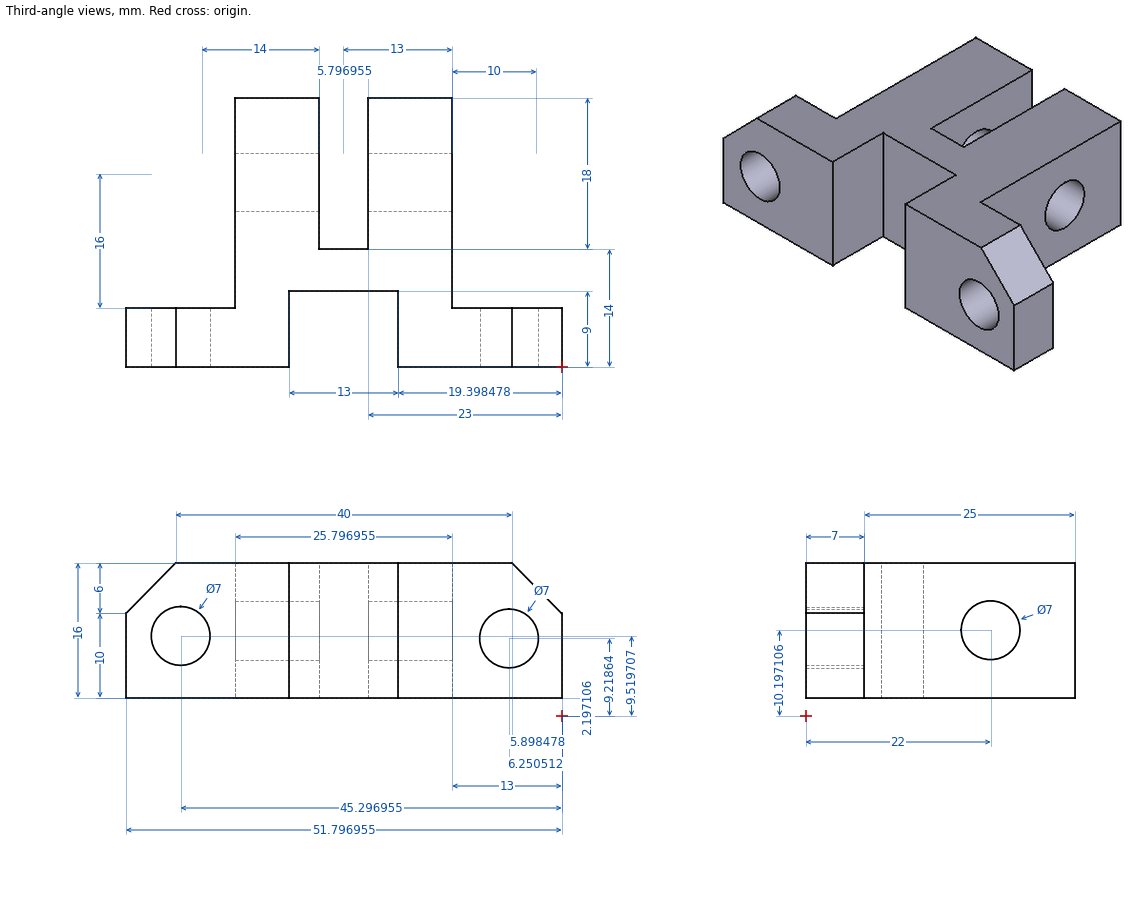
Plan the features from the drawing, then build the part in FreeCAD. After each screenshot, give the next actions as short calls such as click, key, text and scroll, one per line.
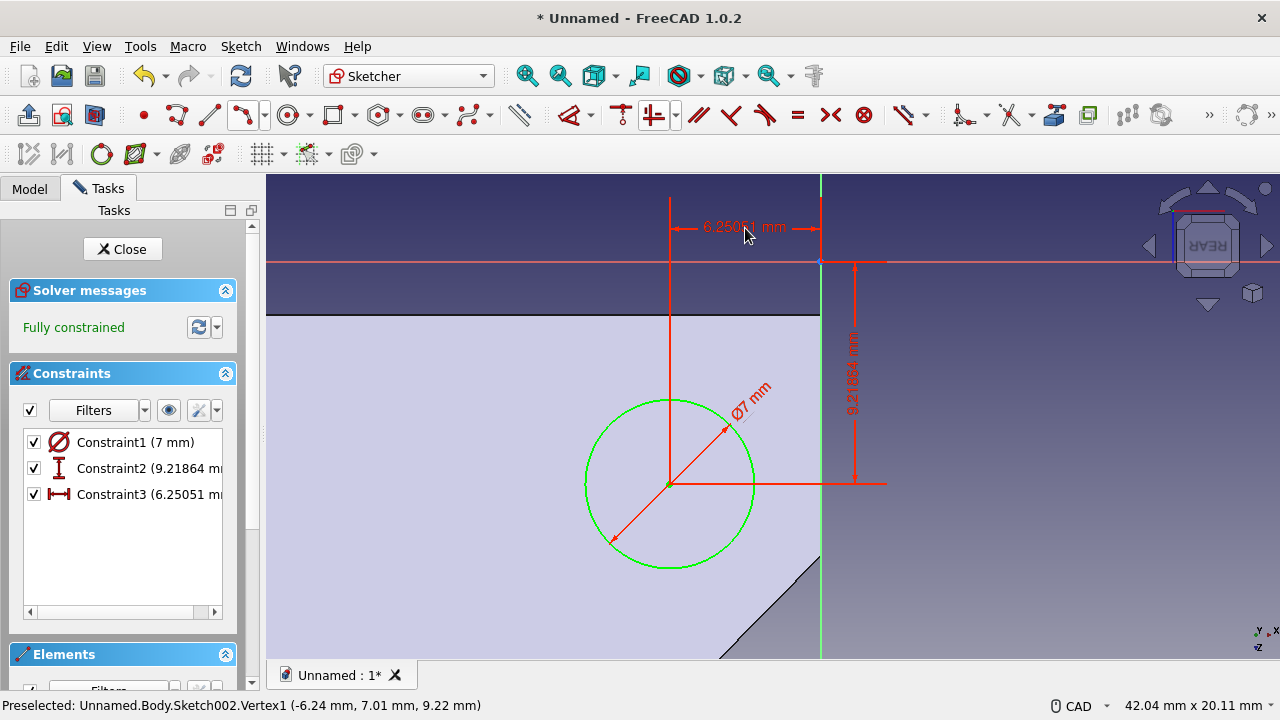
click(123, 249)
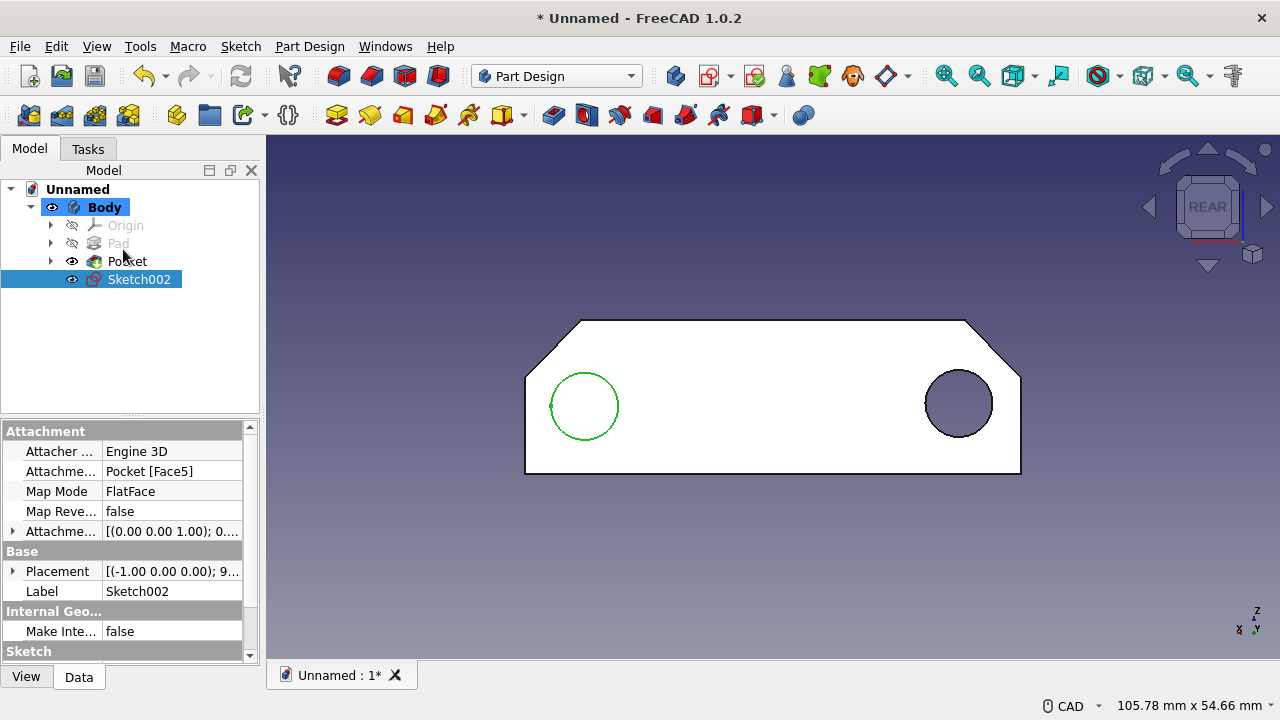
click(554, 116)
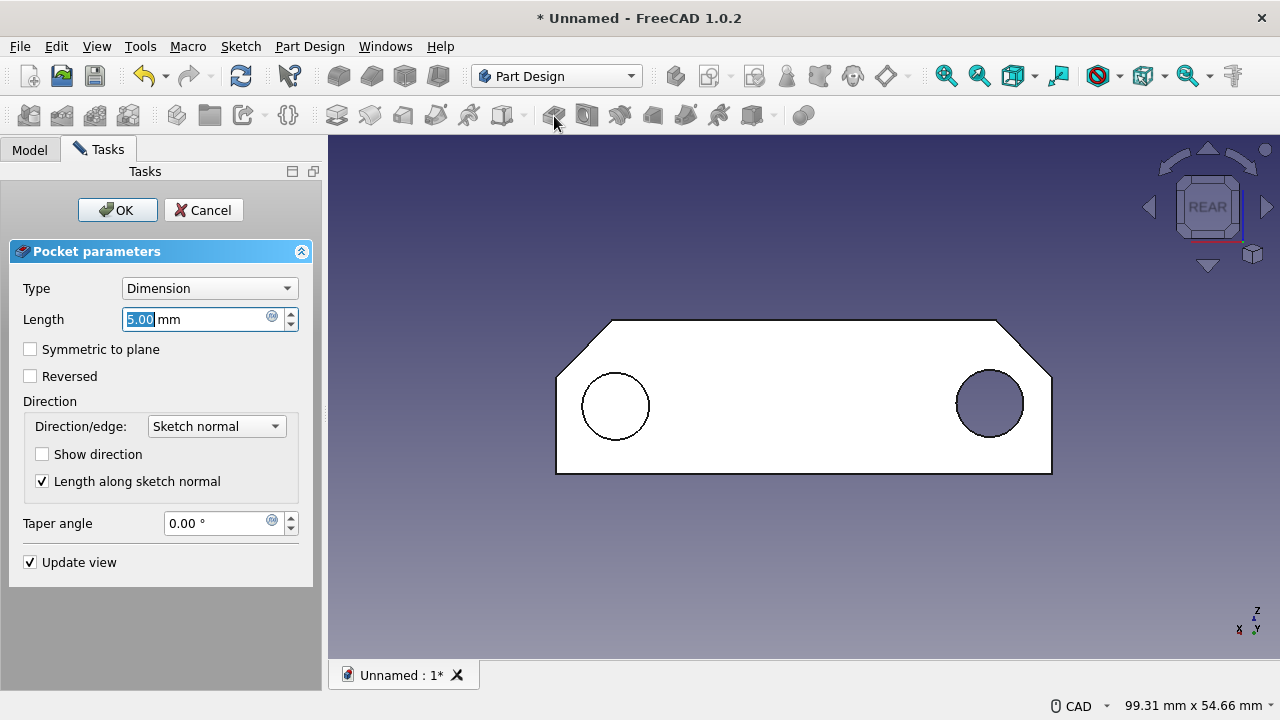
click(210, 288)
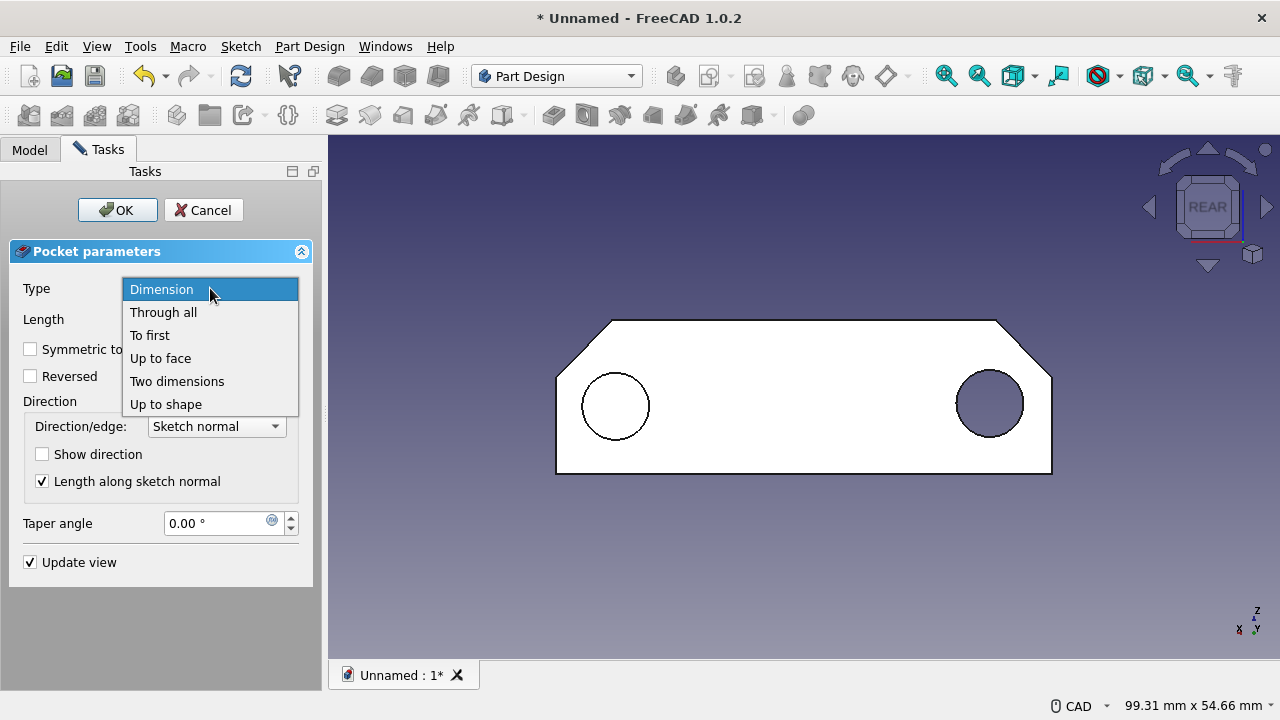
click(208, 382)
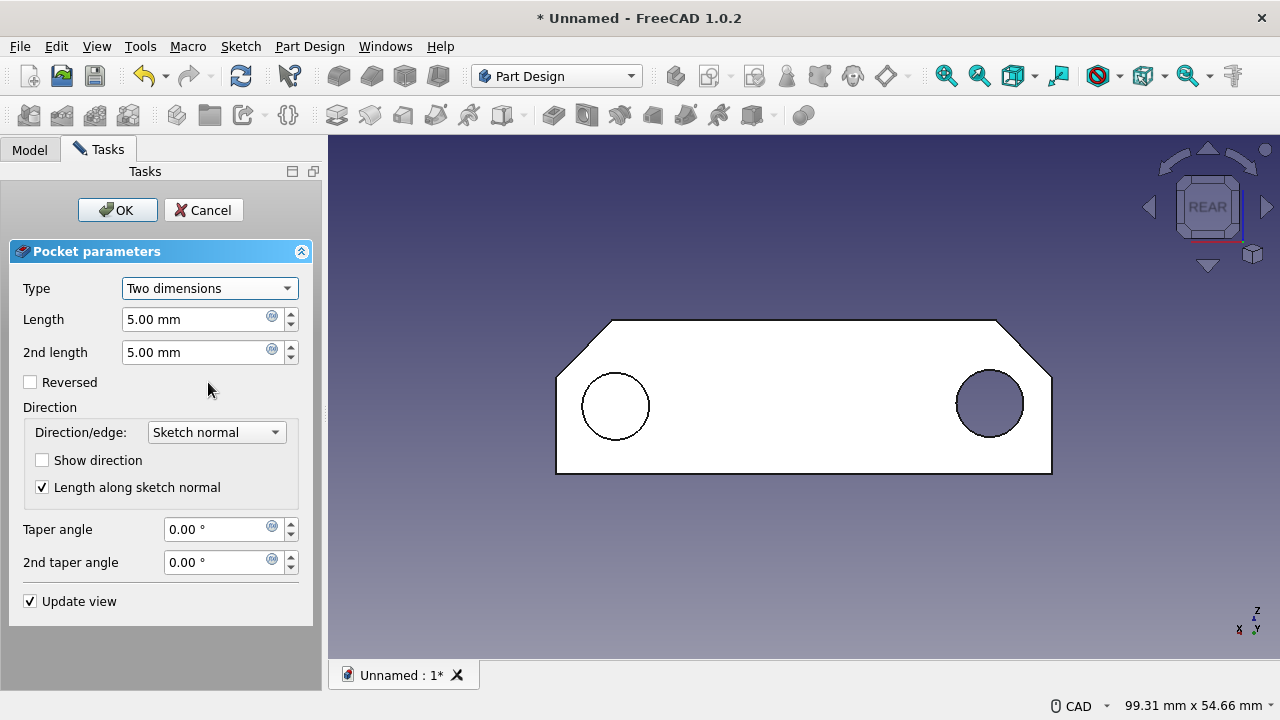
triple_click(204, 320)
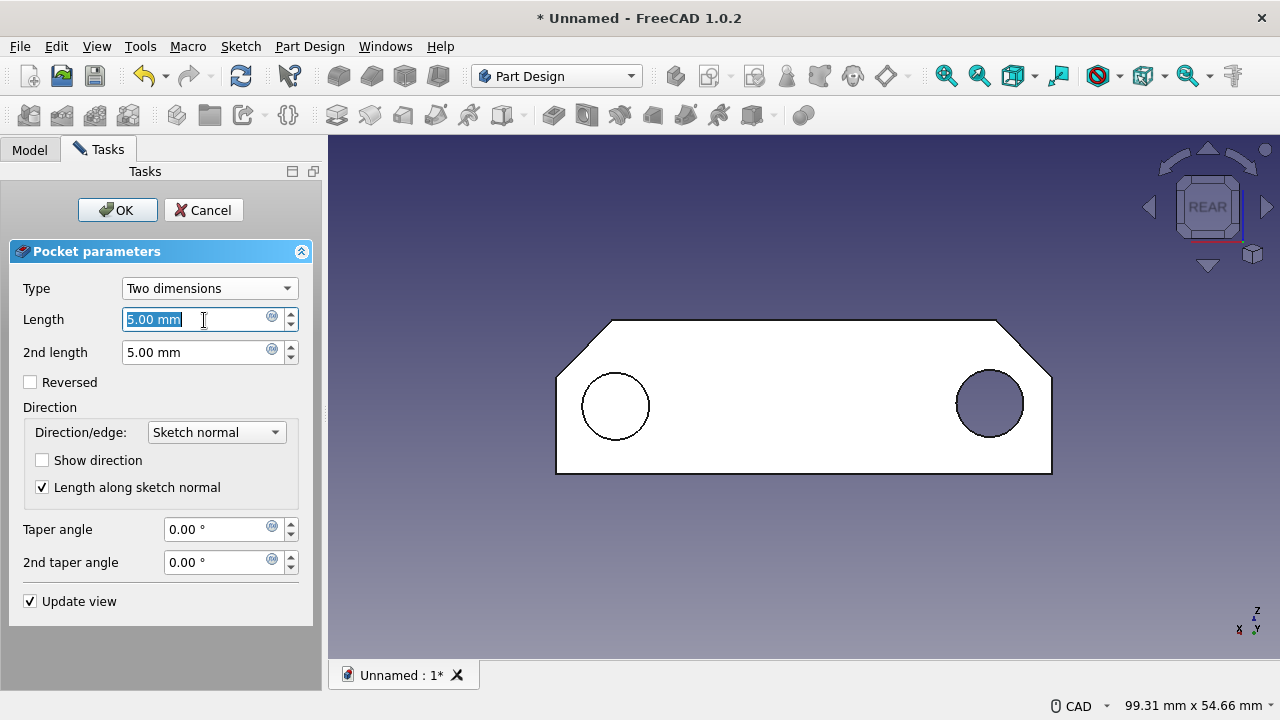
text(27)
key(Tab)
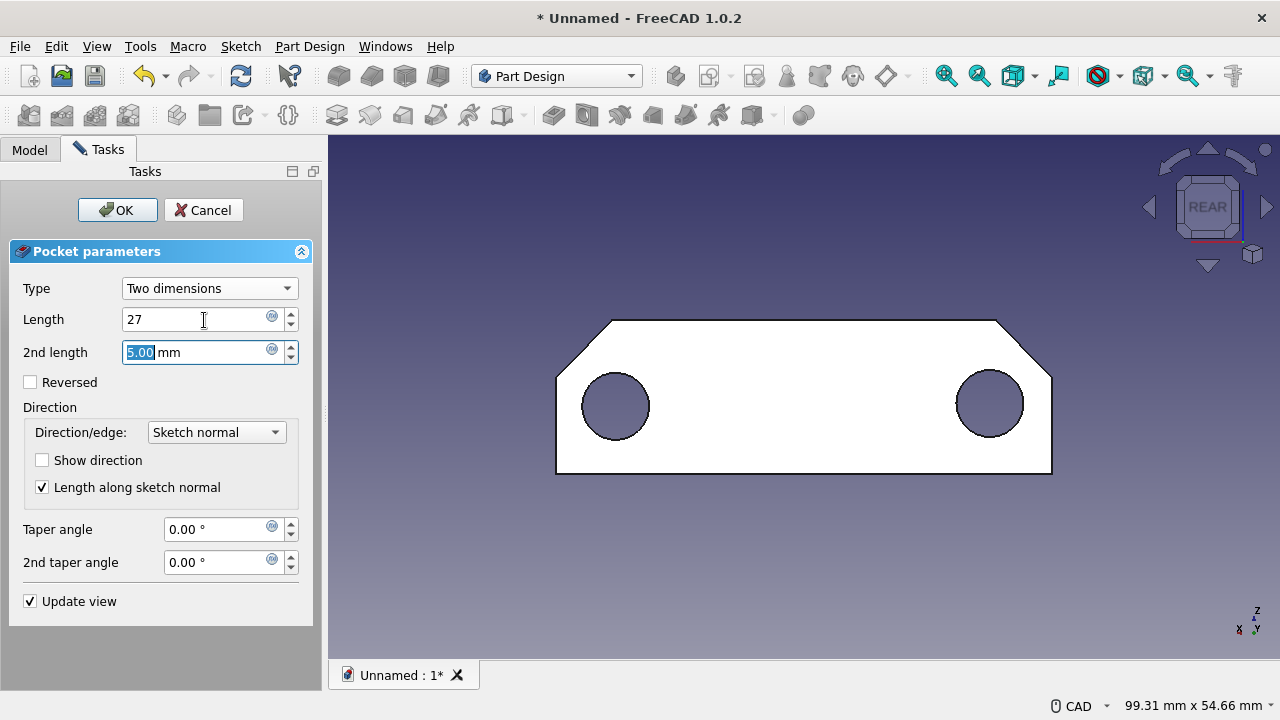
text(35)
key(Tab)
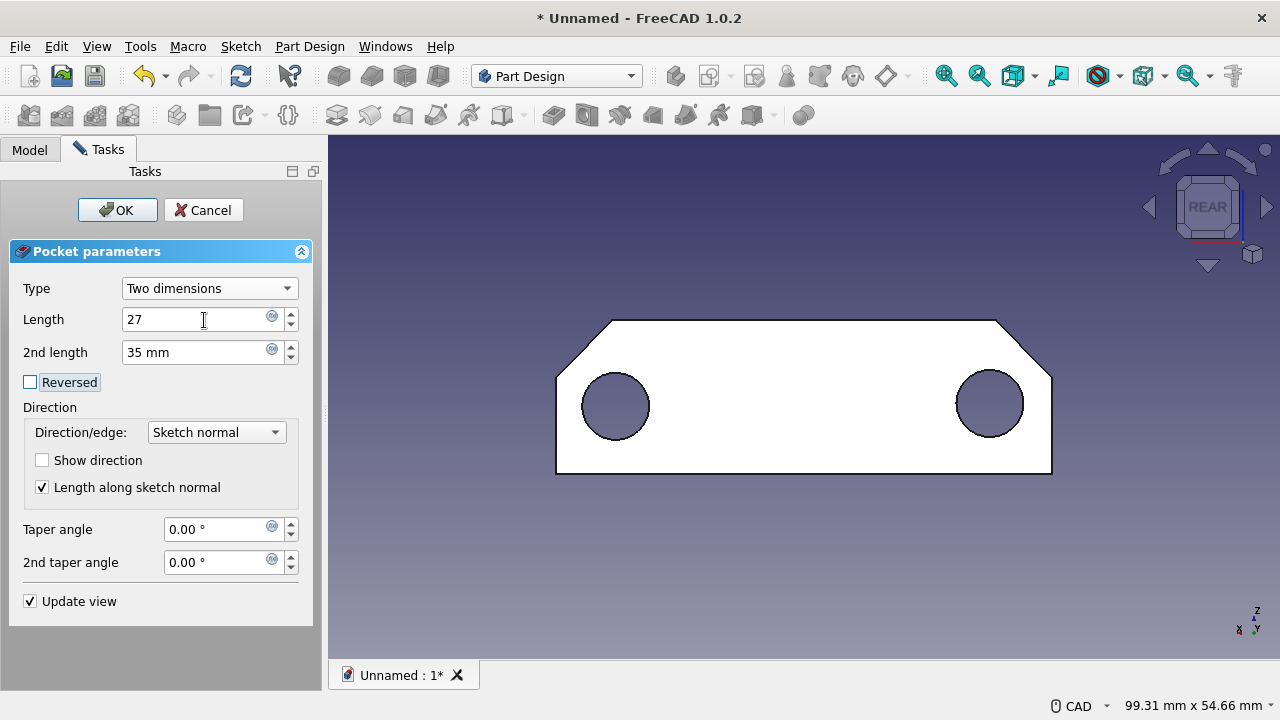
click(31, 382)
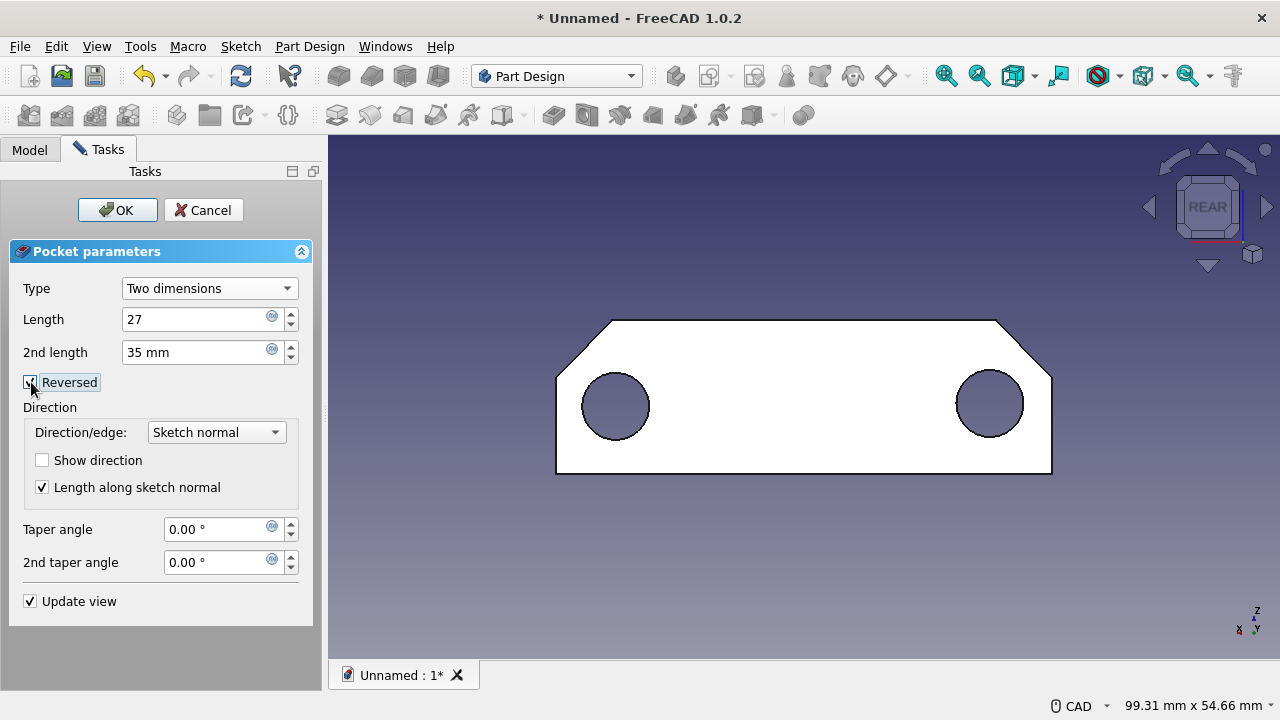
click(118, 210)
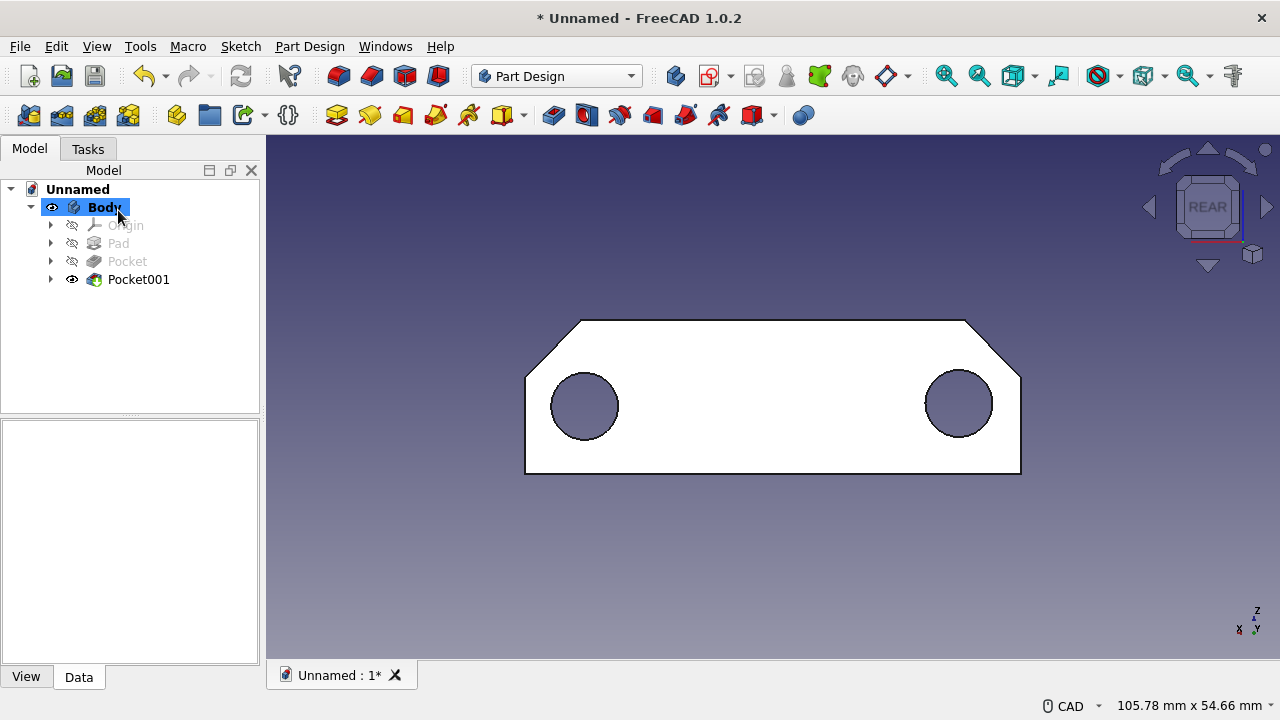
click(702, 396)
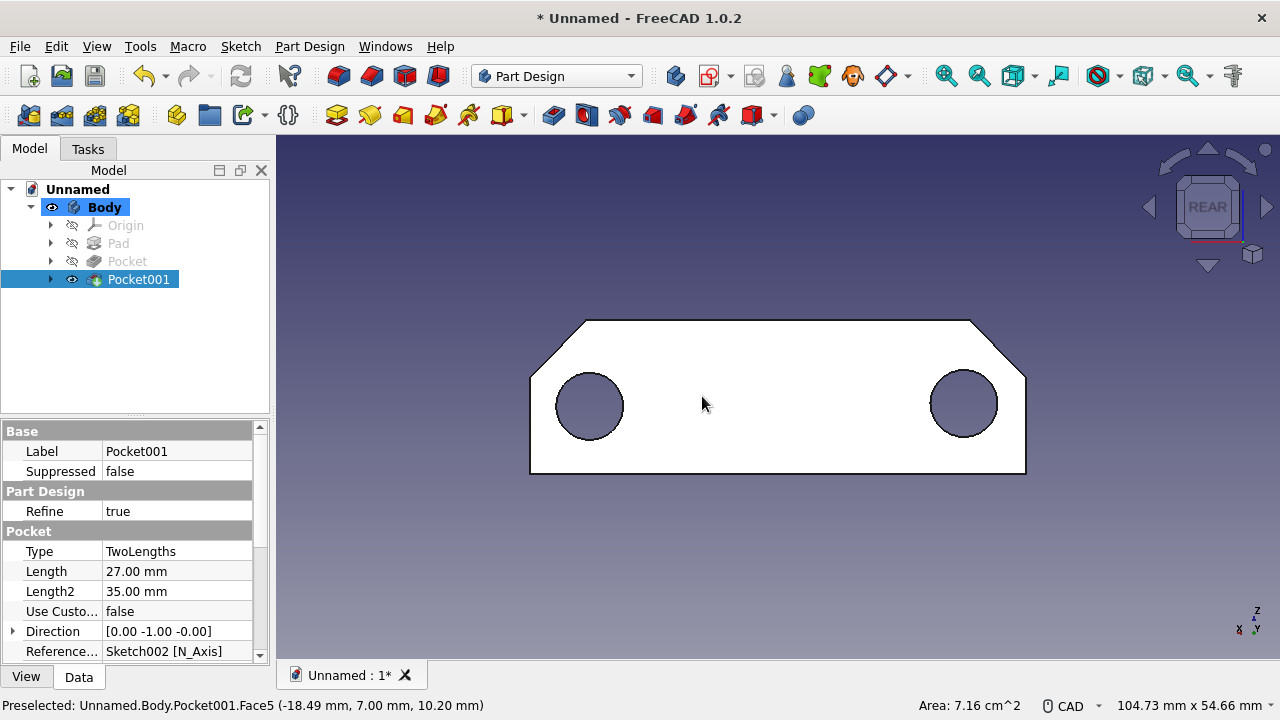
click(708, 76)